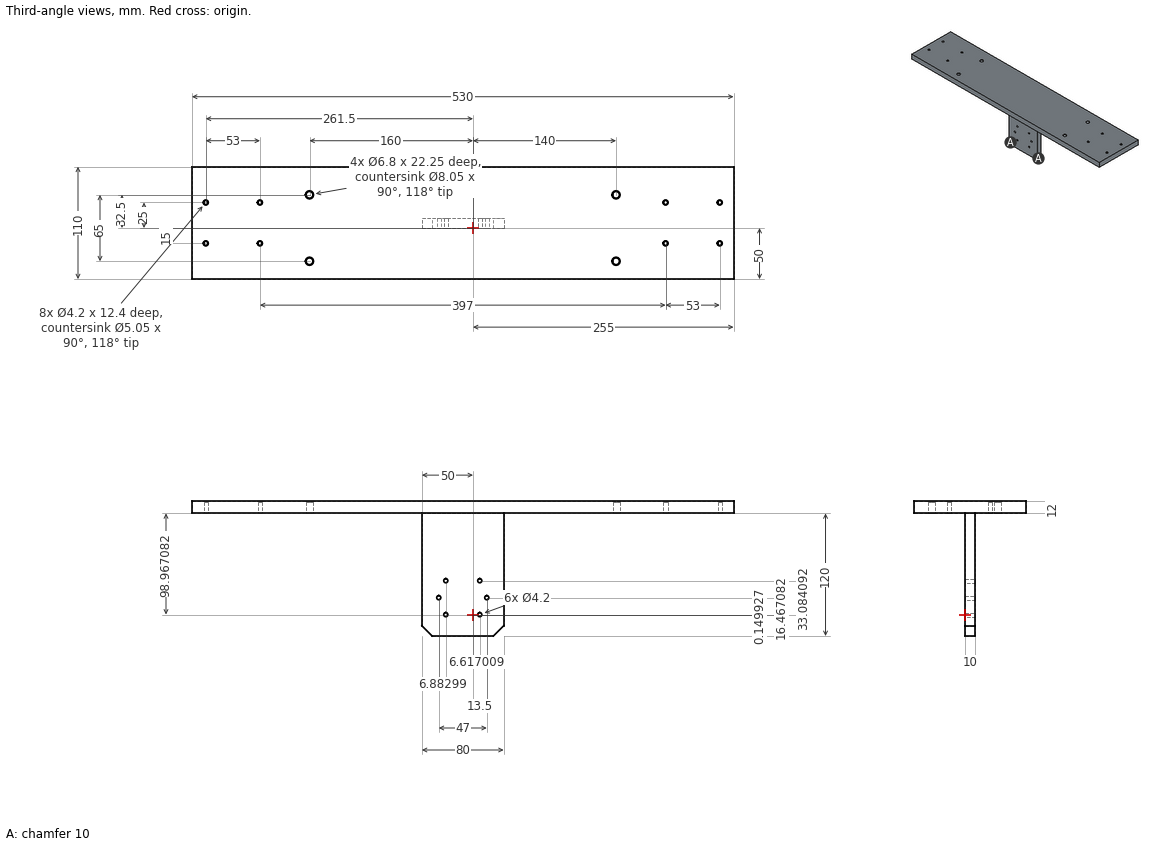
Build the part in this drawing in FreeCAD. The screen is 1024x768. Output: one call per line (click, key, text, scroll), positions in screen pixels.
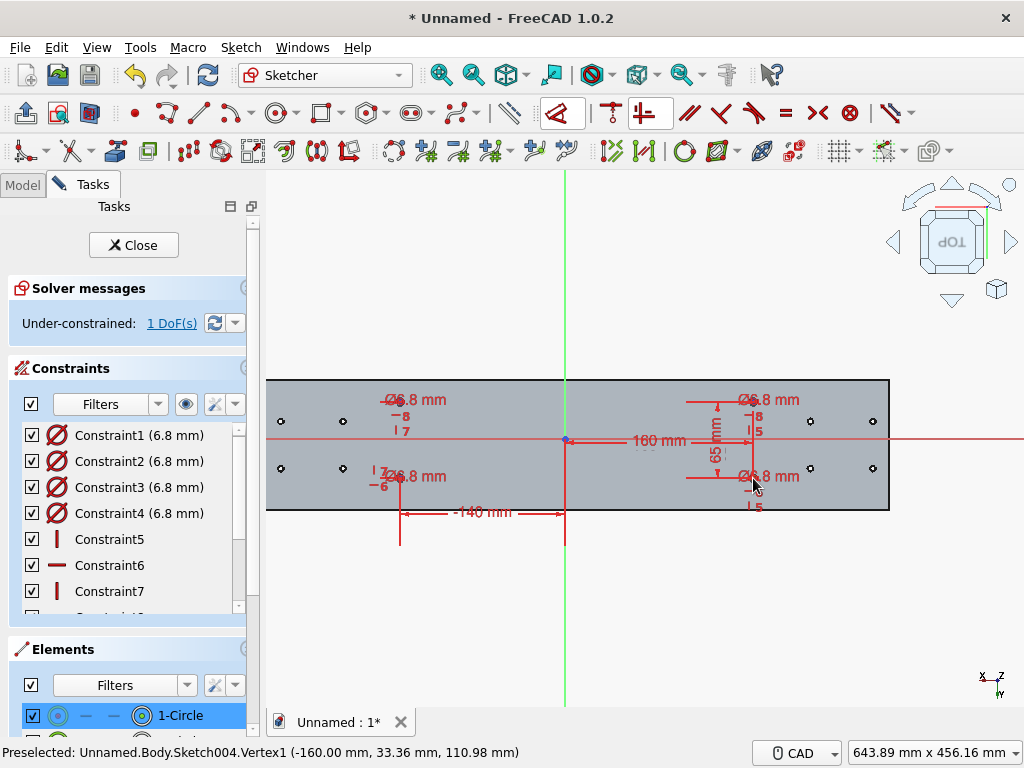
key(i)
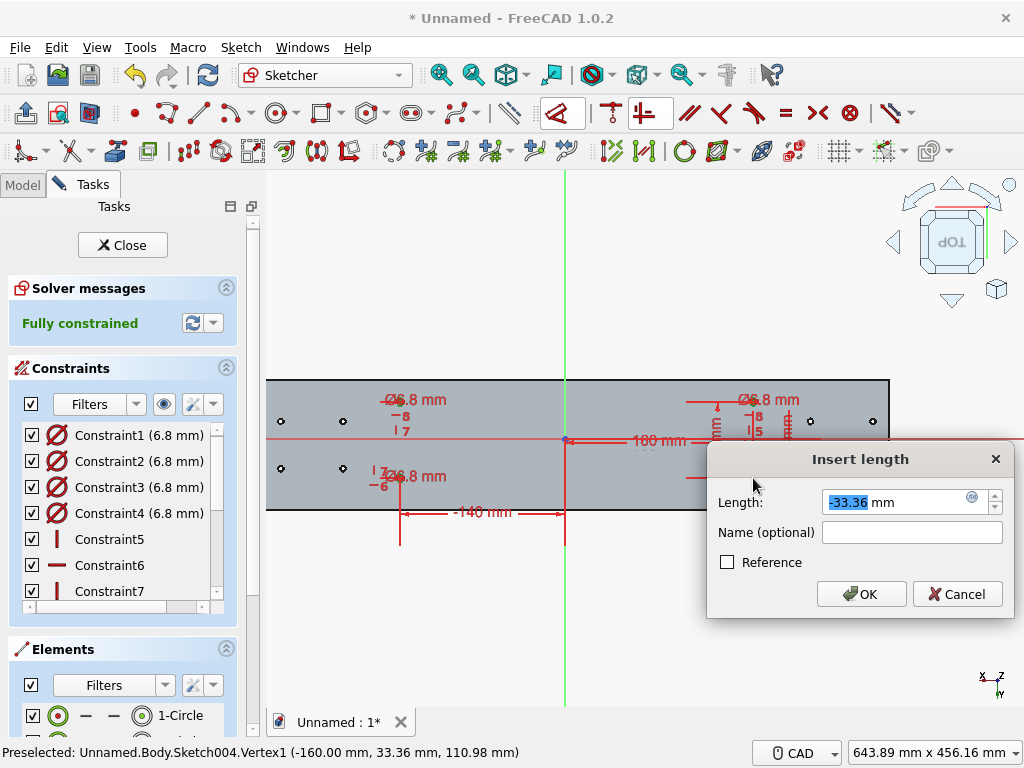
text(-32.5)
key(Return)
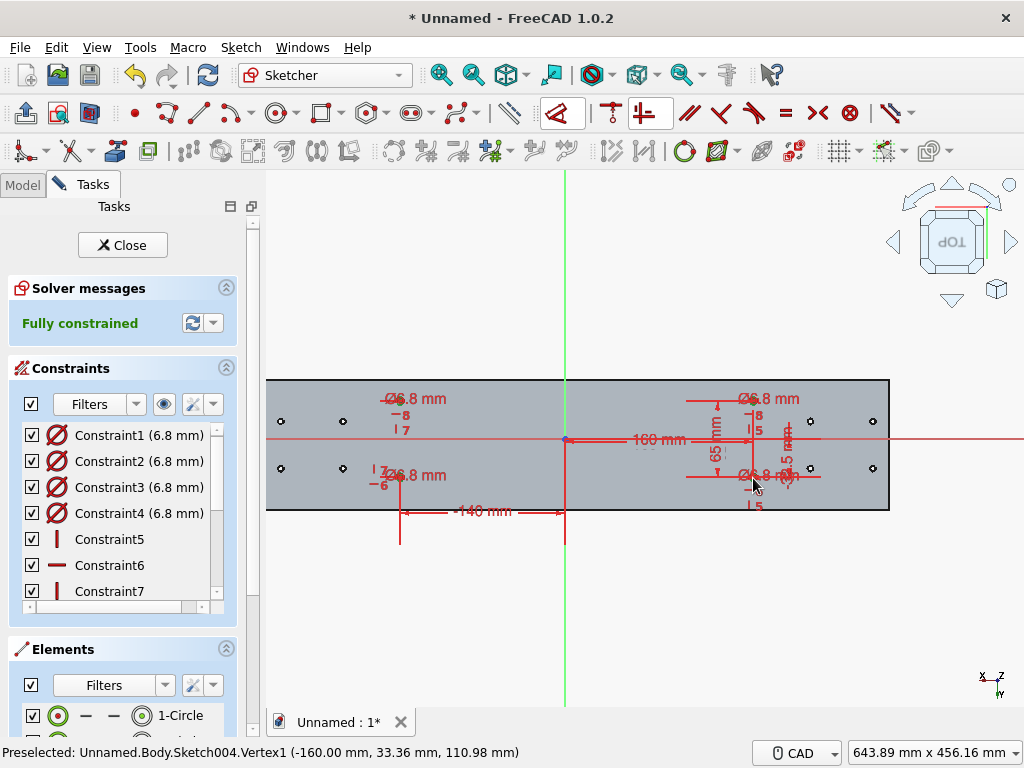
click(123, 245)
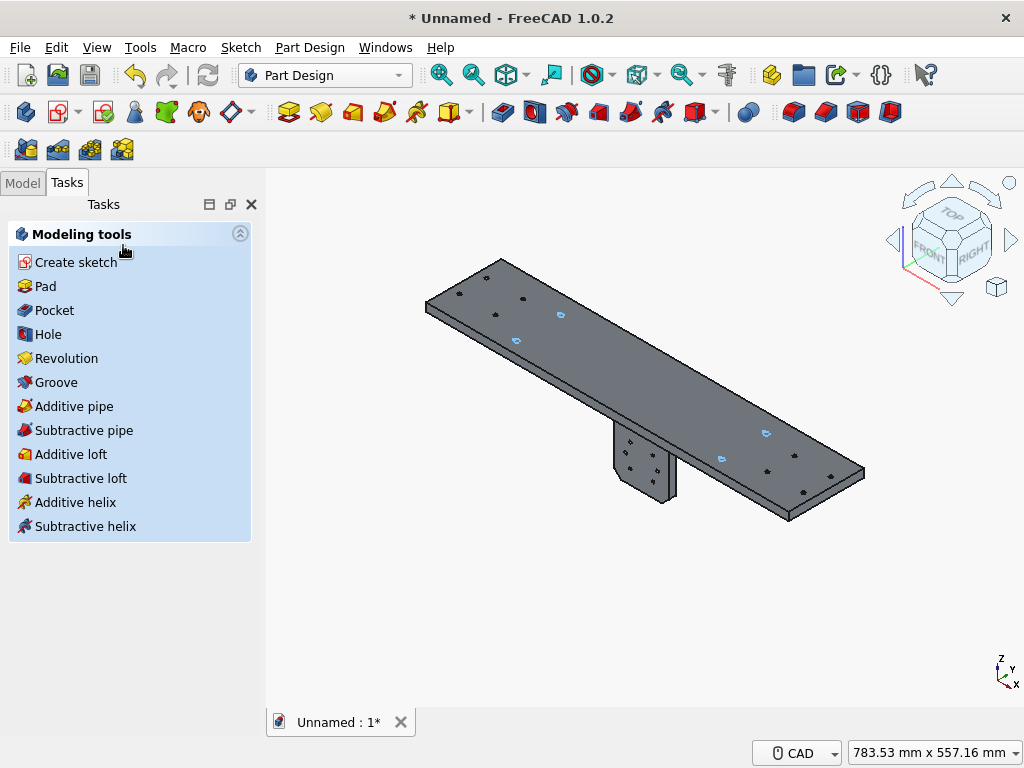
click(536, 112)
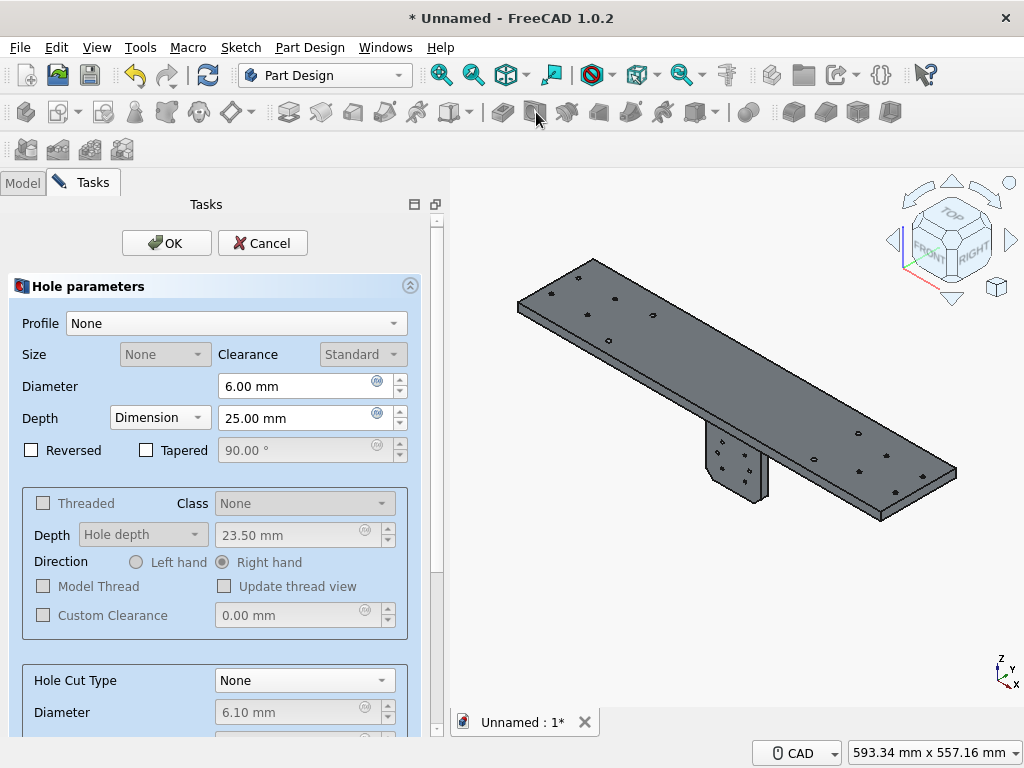
triple_click(305, 386)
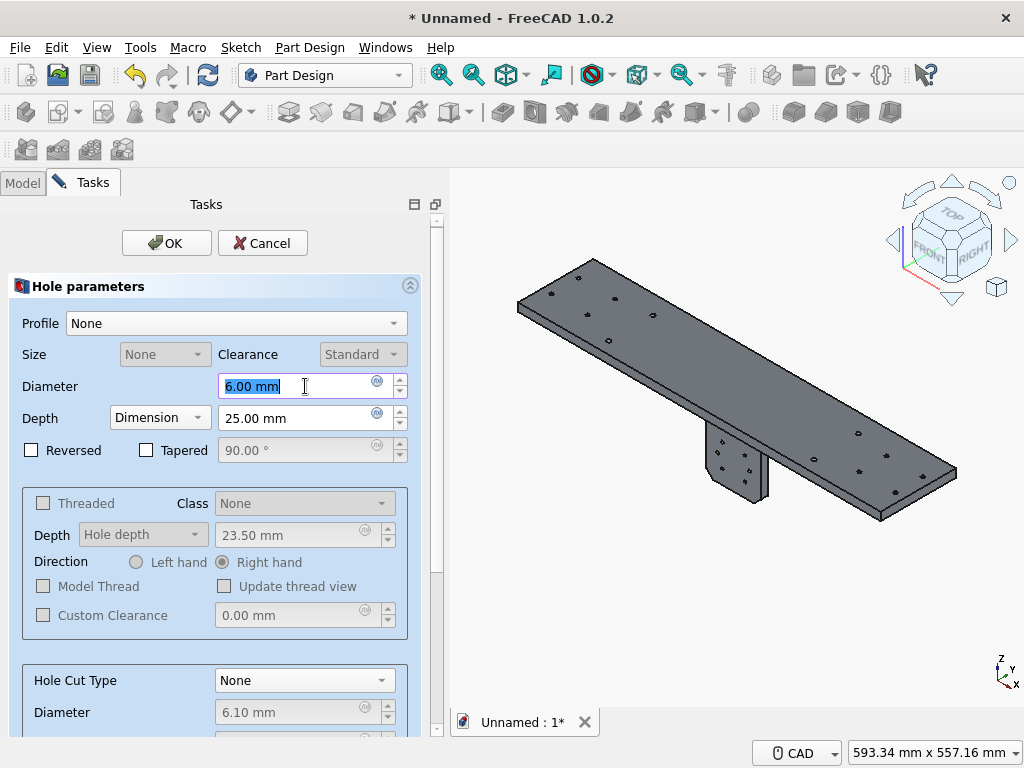
text(6.8)
key(Tab)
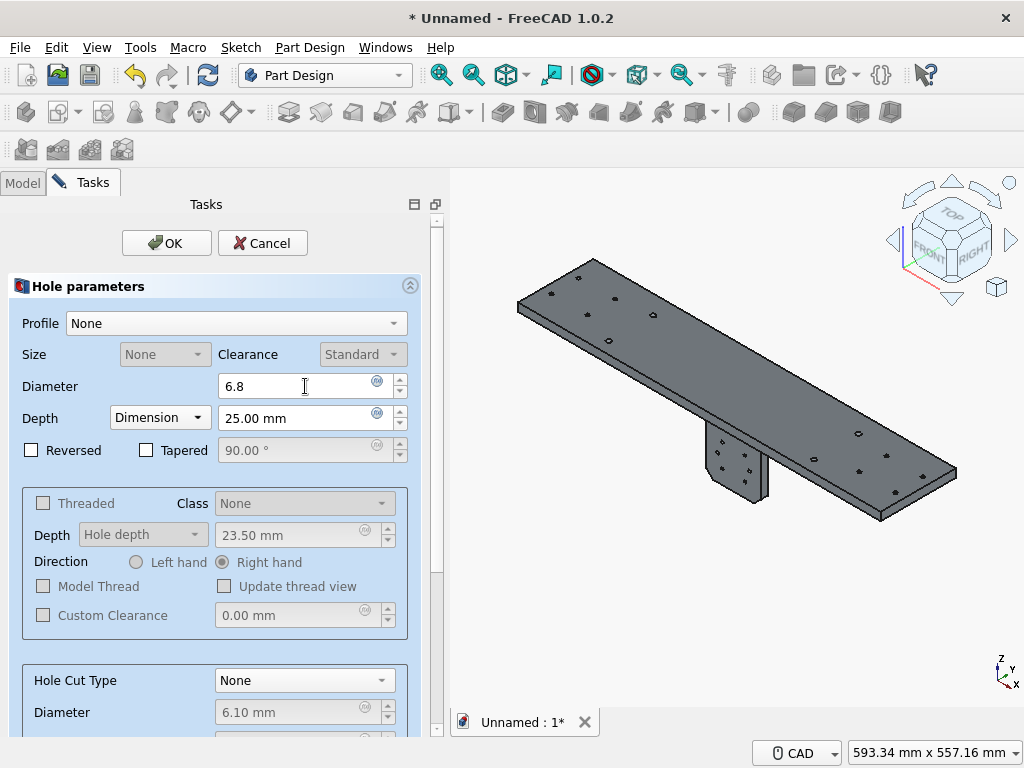
triple_click(305, 418)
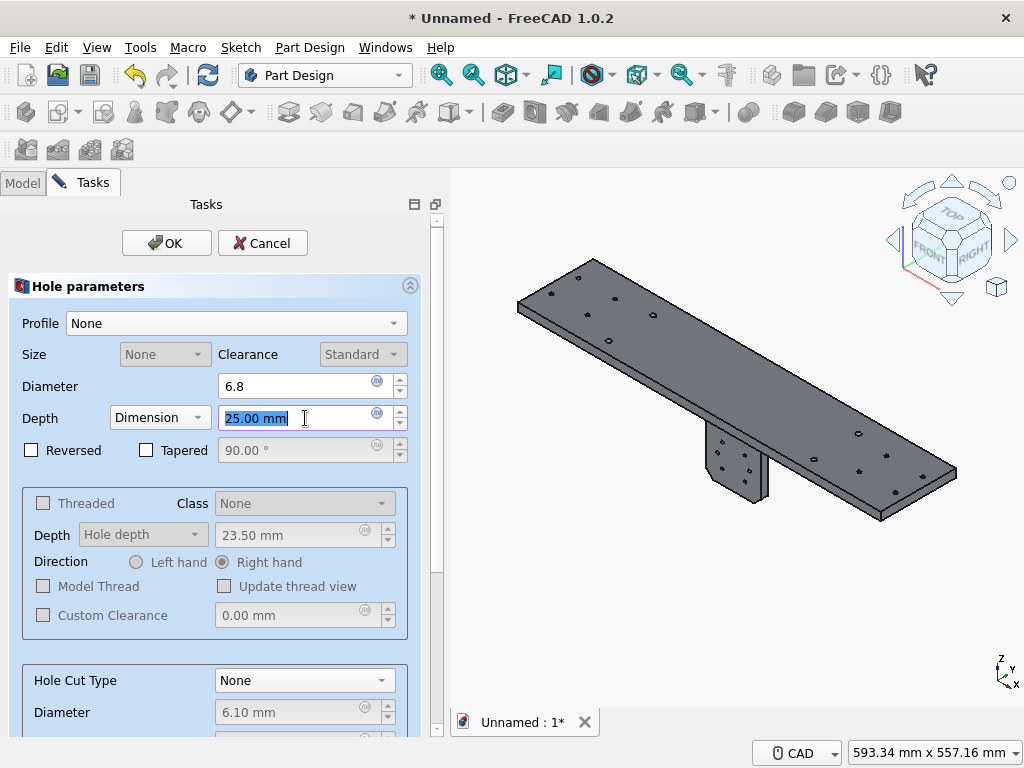
text(22.25)
key(Tab)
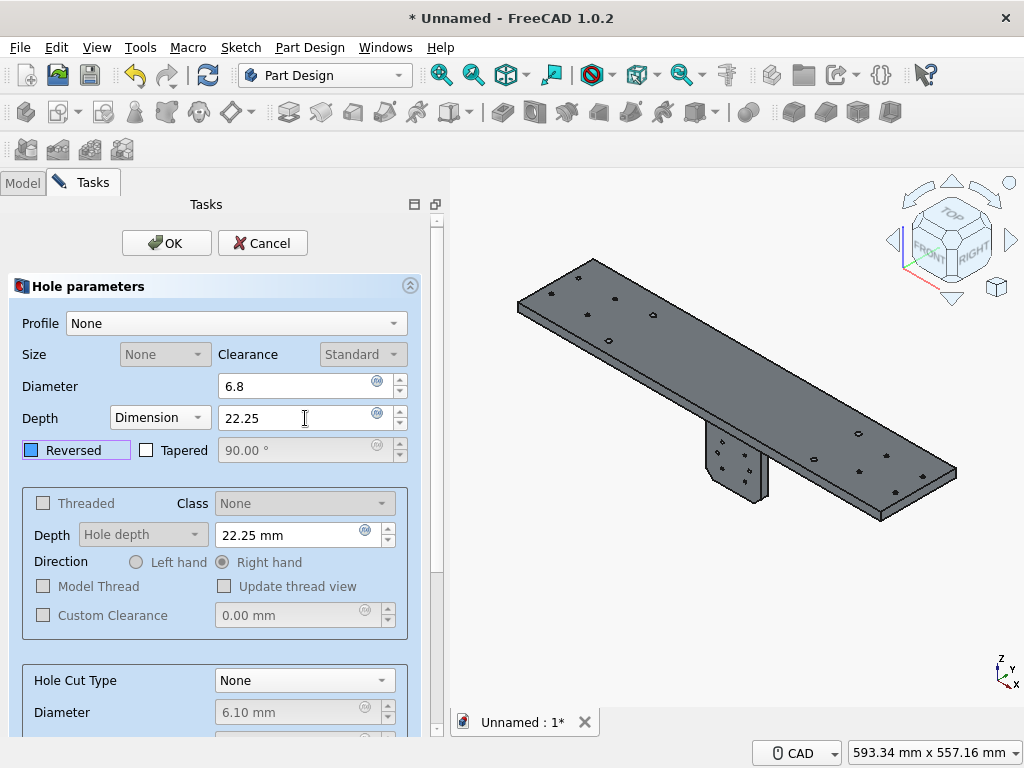
click(306, 680)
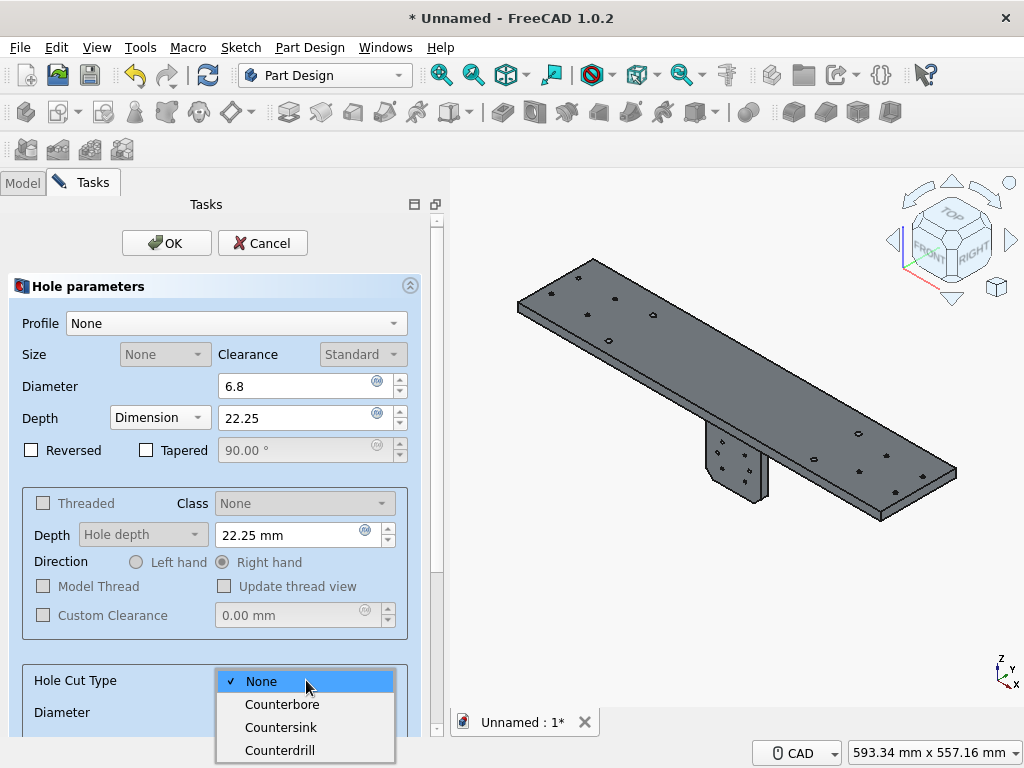
click(304, 728)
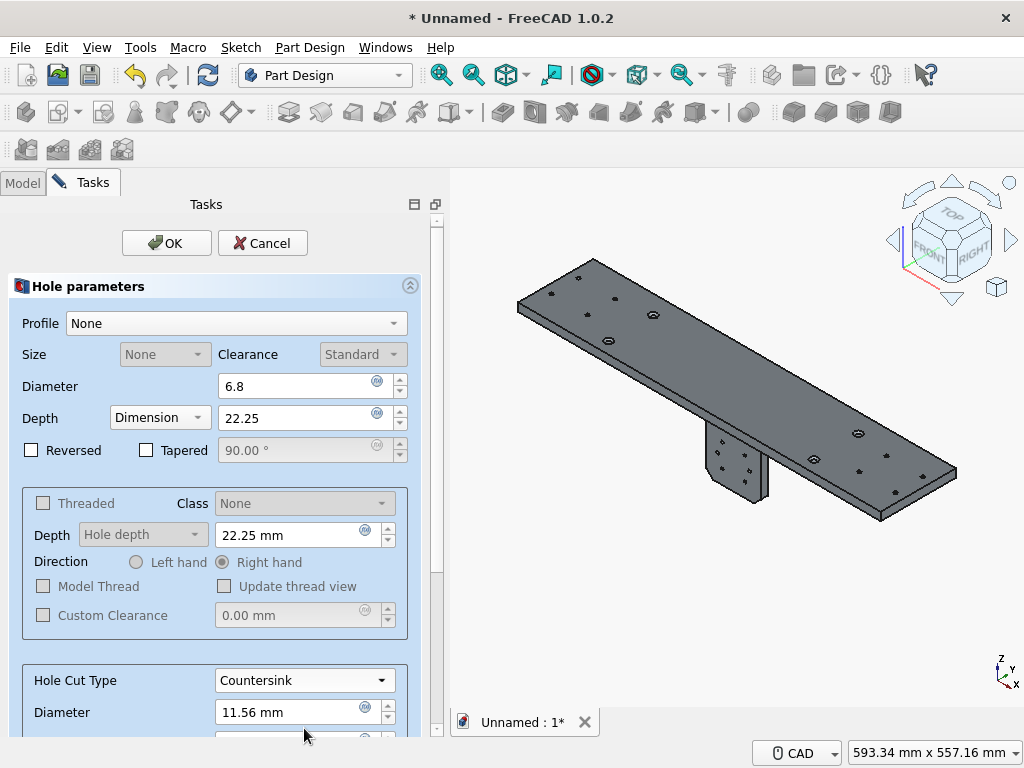
triple_click(298, 712)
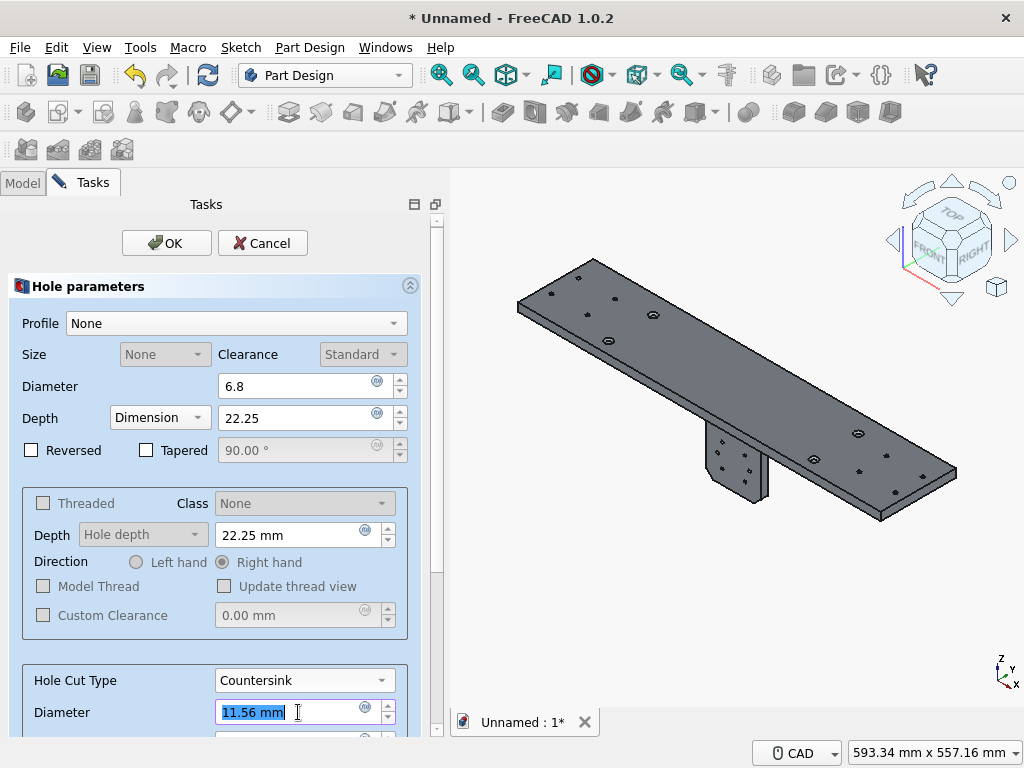
text(8.05)
key(Tab)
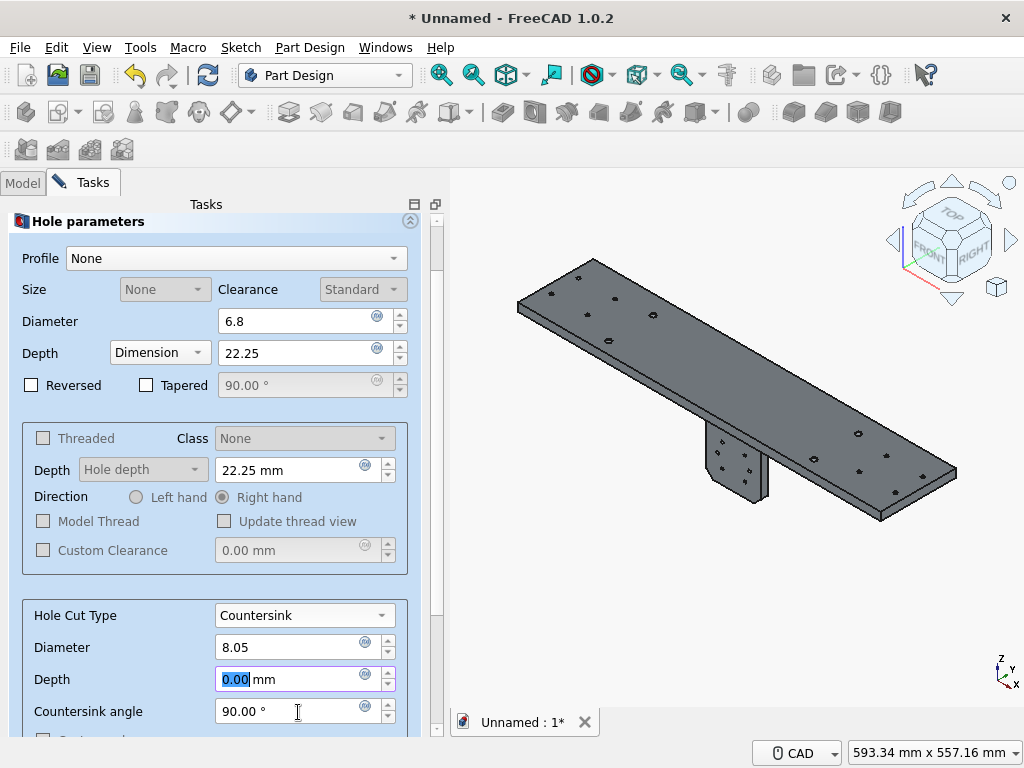
scroll(437, 475, up, 2)